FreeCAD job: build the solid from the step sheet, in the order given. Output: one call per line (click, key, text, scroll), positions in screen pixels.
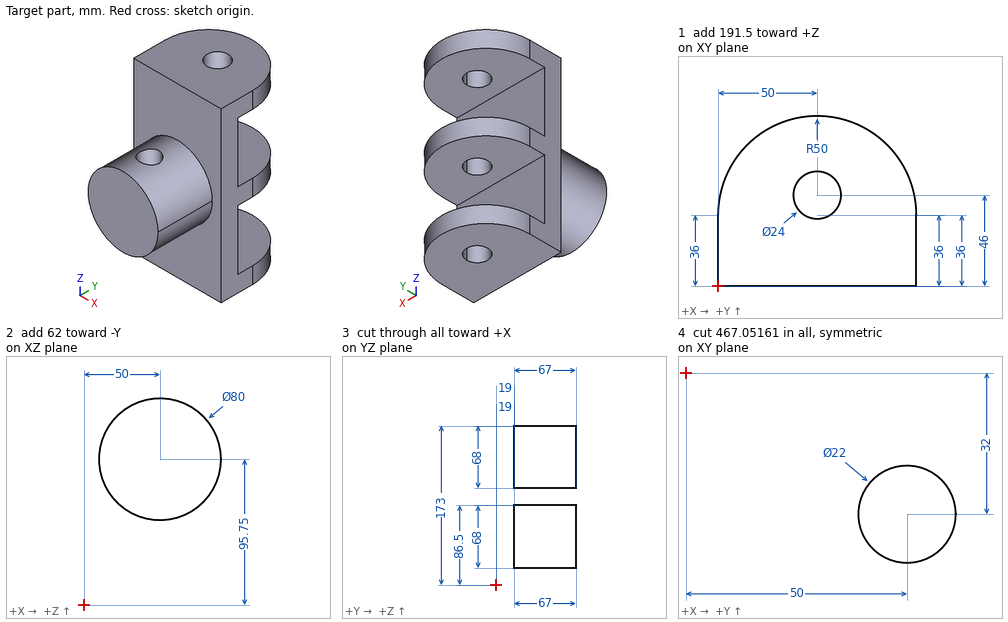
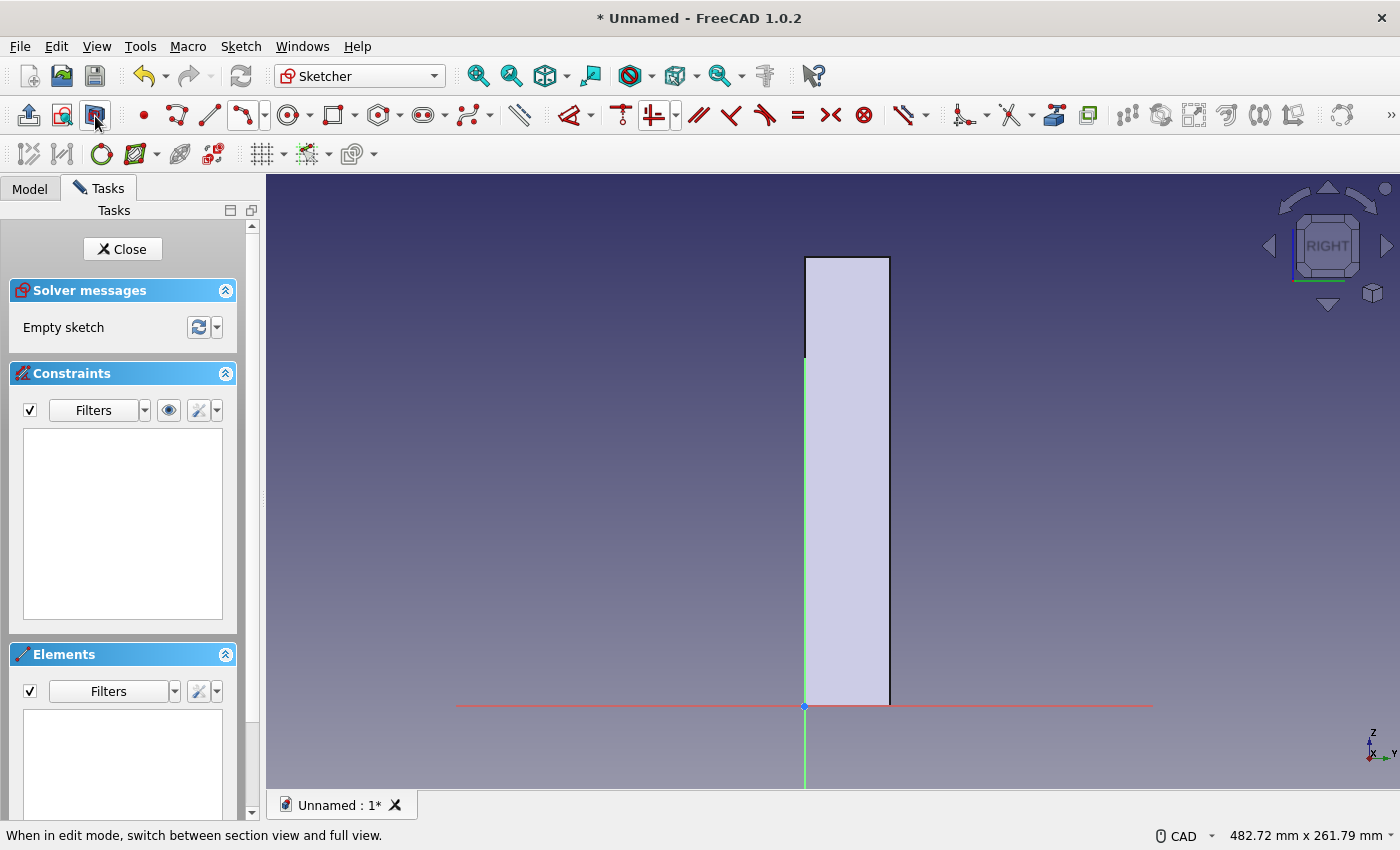
click(332, 116)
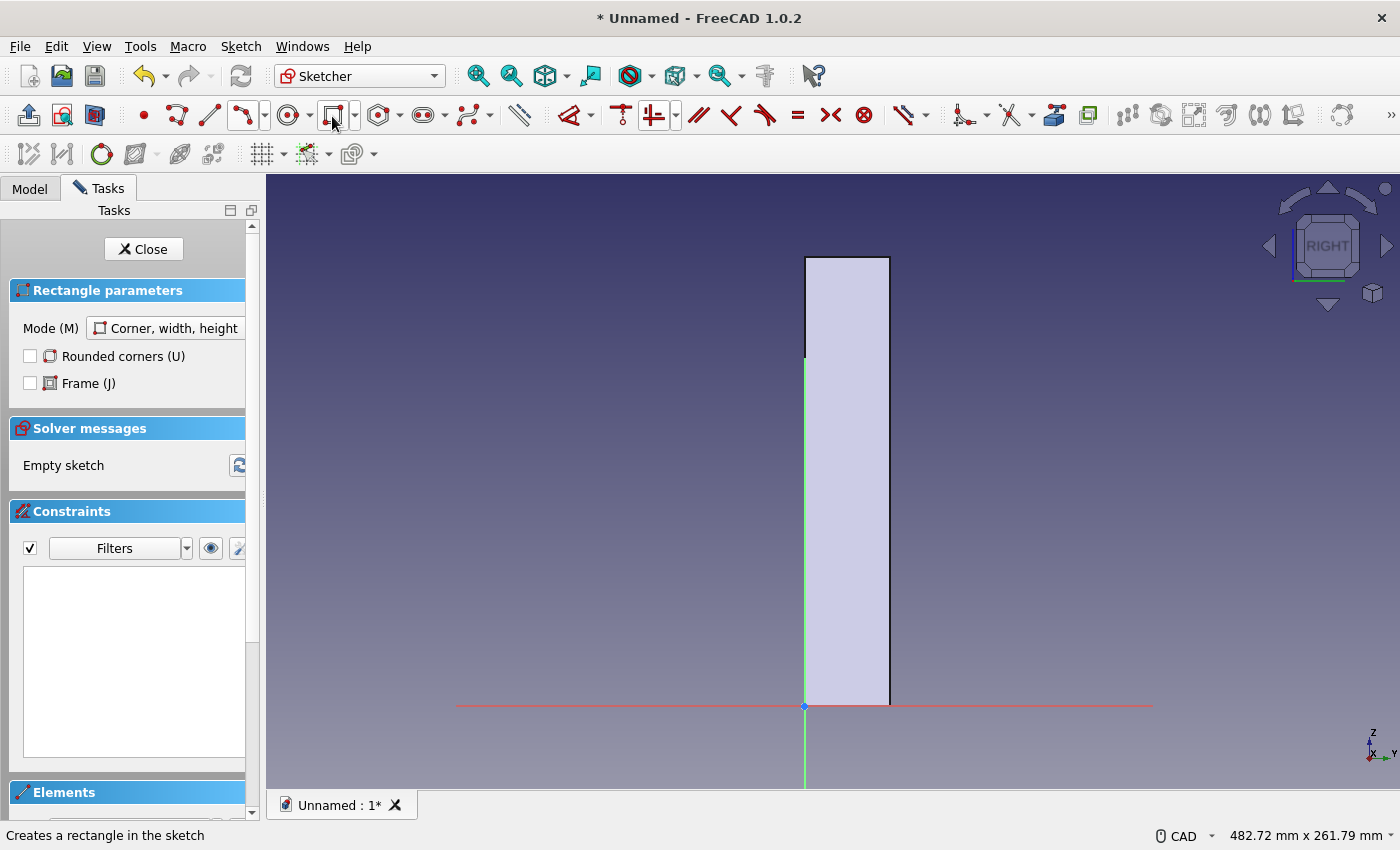
click(850, 503)
click(1007, 663)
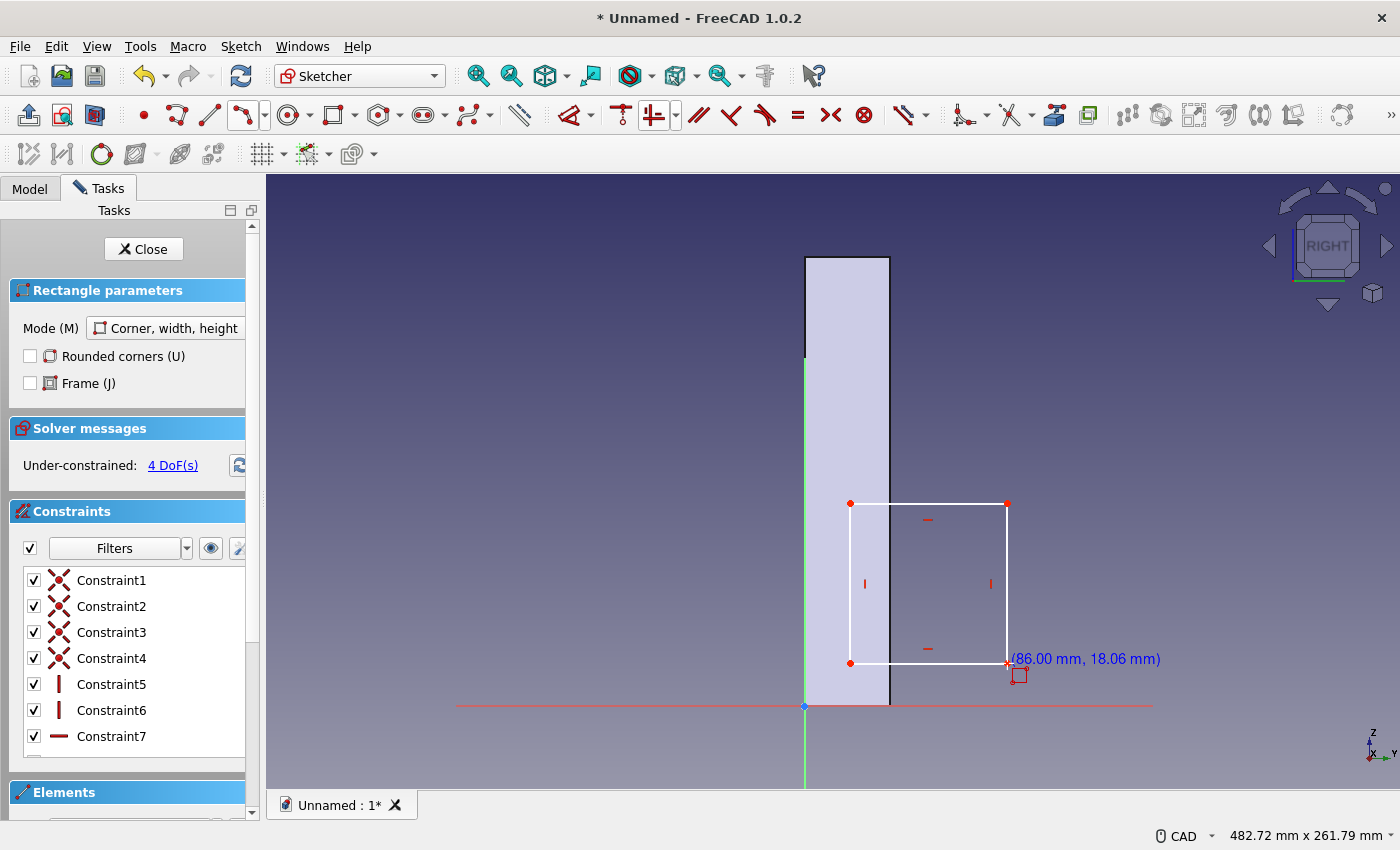
click(850, 300)
click(1007, 460)
key(Escape)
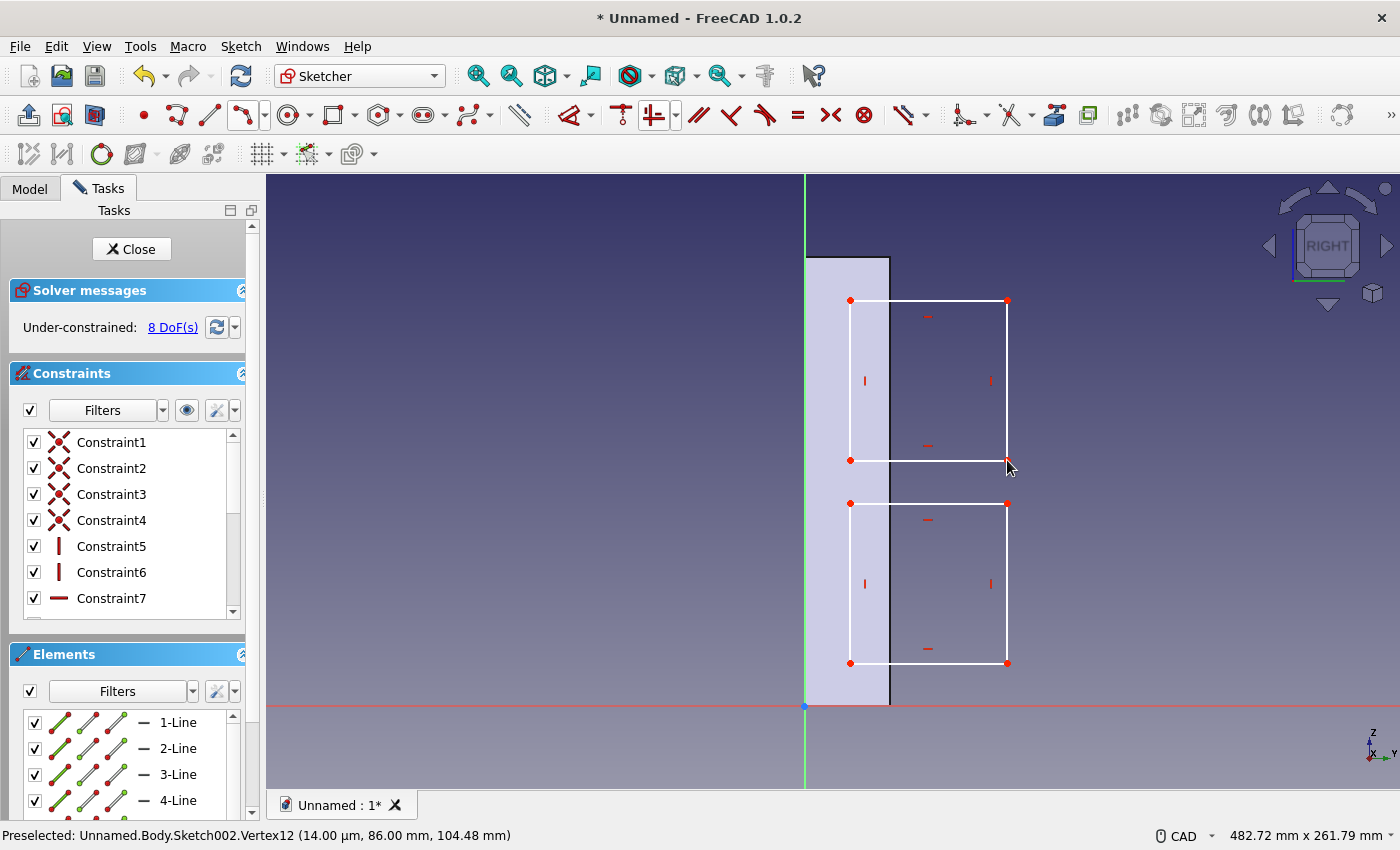
click(568, 116)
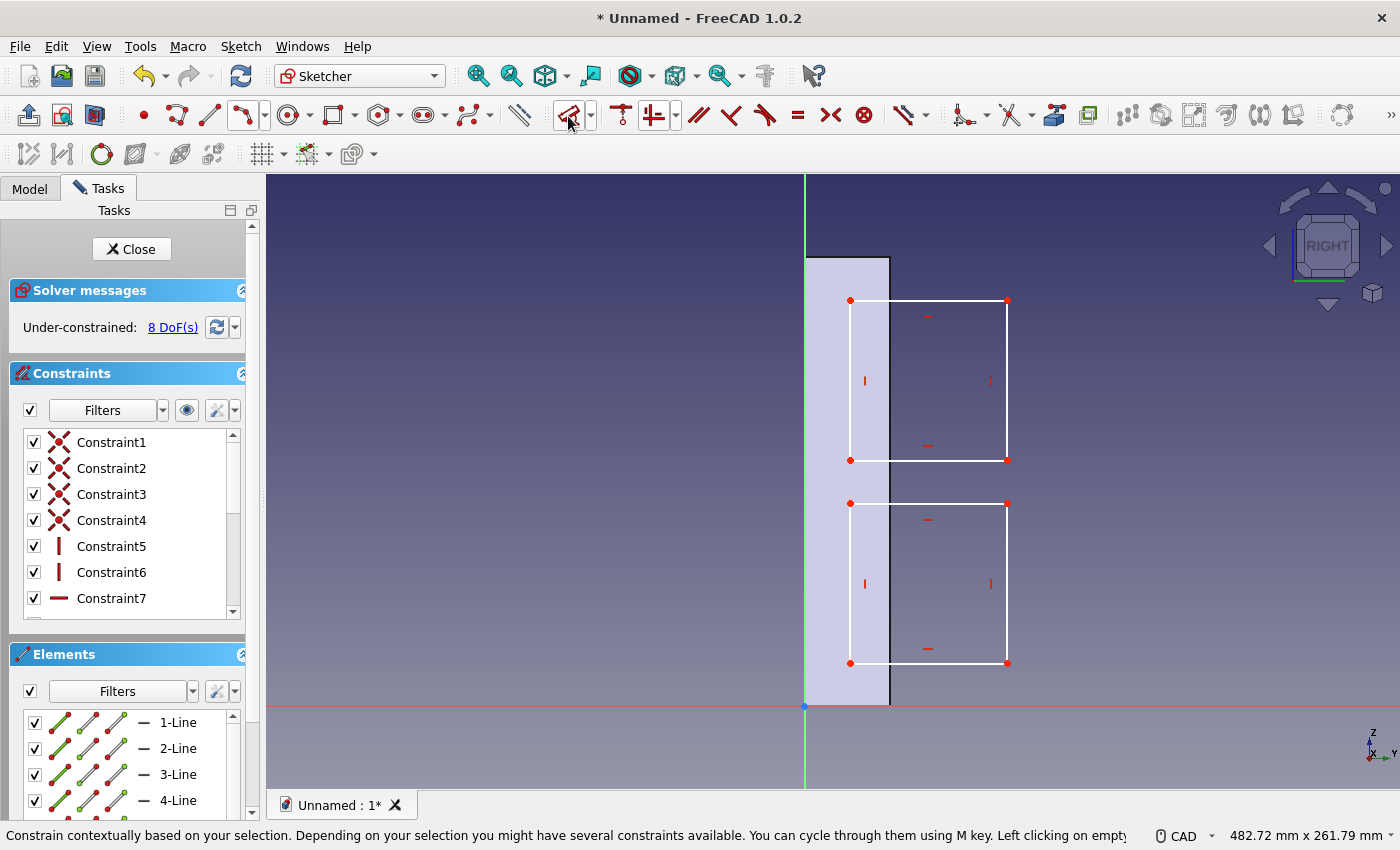
click(850, 552)
click(884, 584)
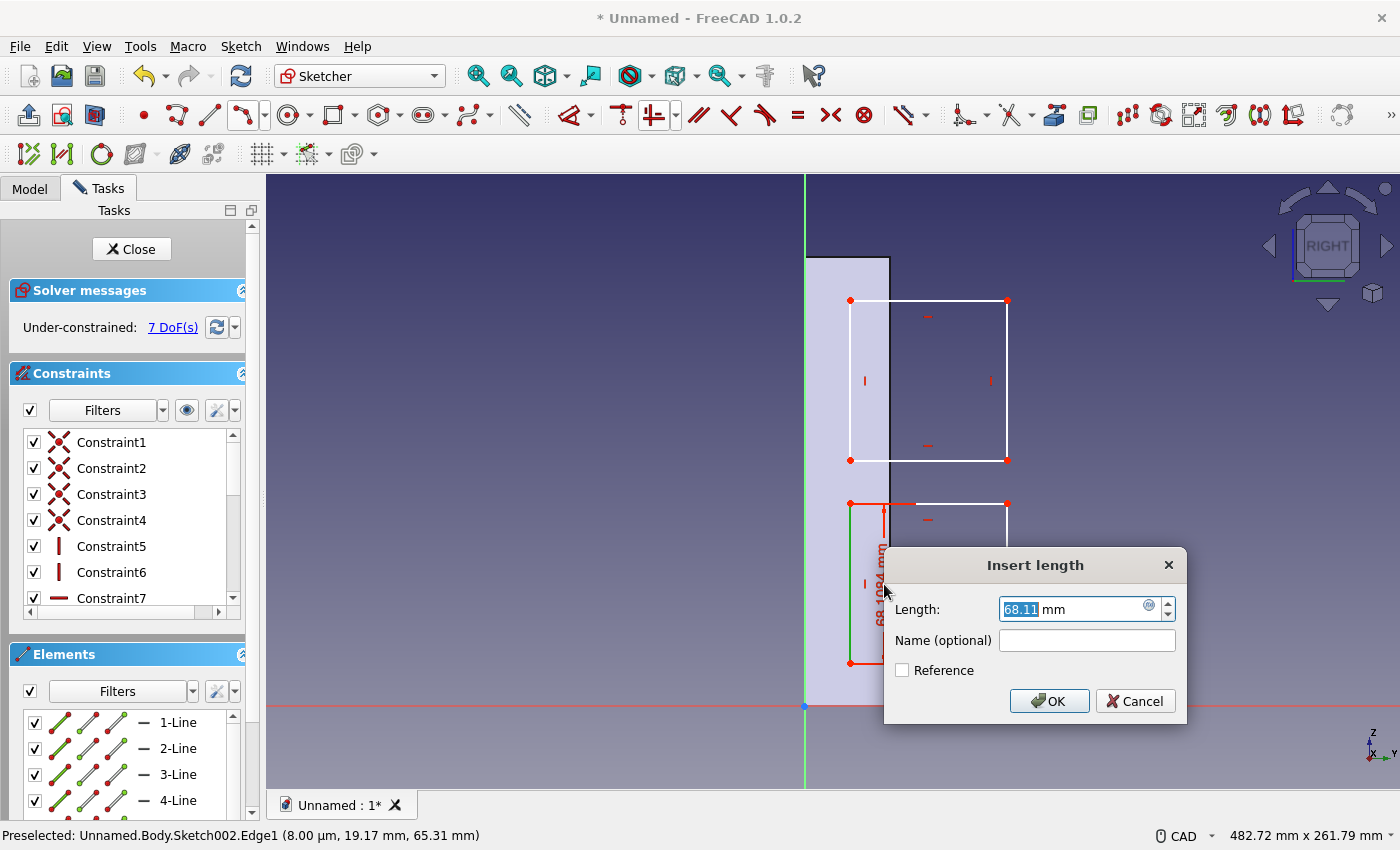
text(68)
key(Return)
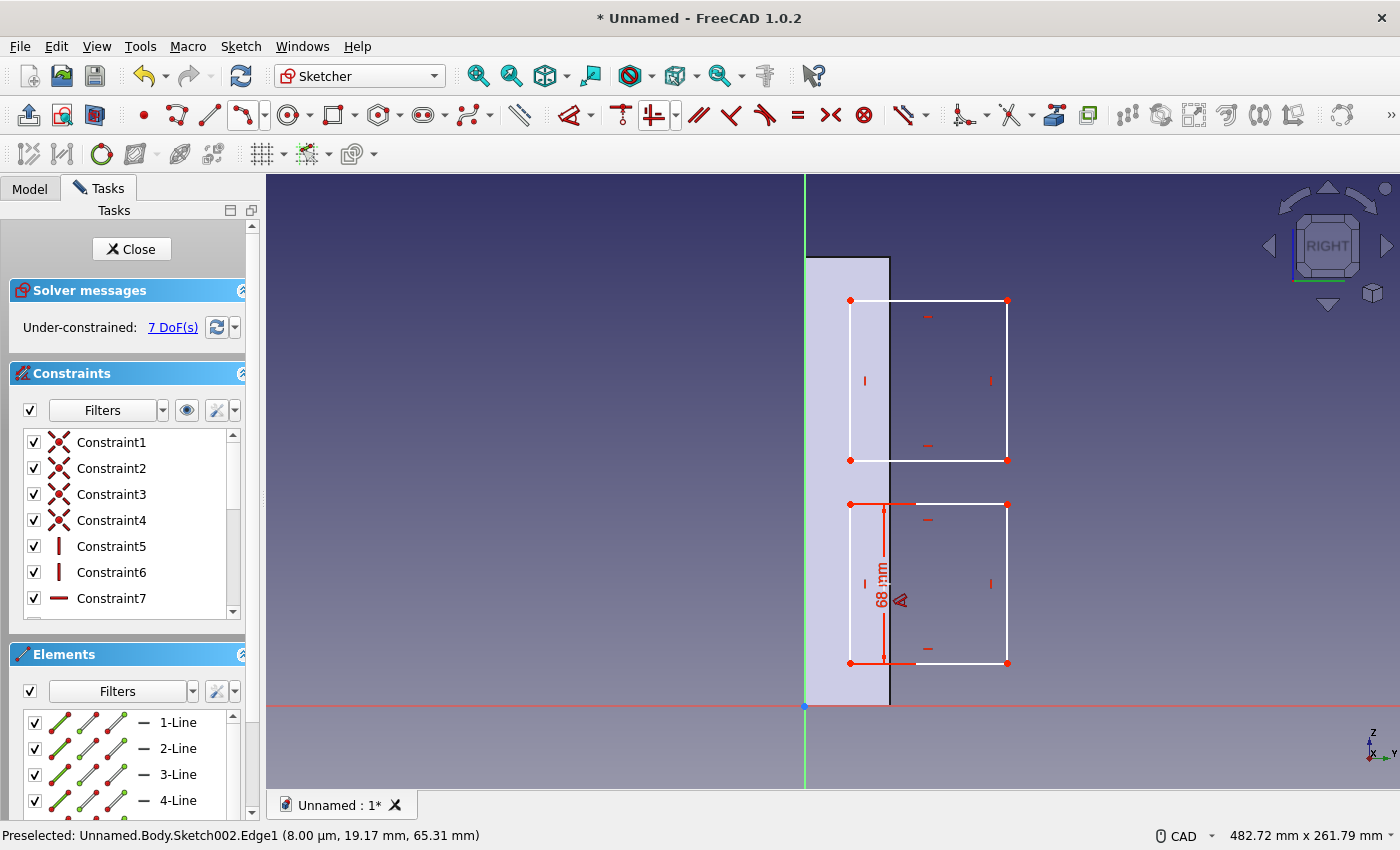
click(897, 664)
click(929, 630)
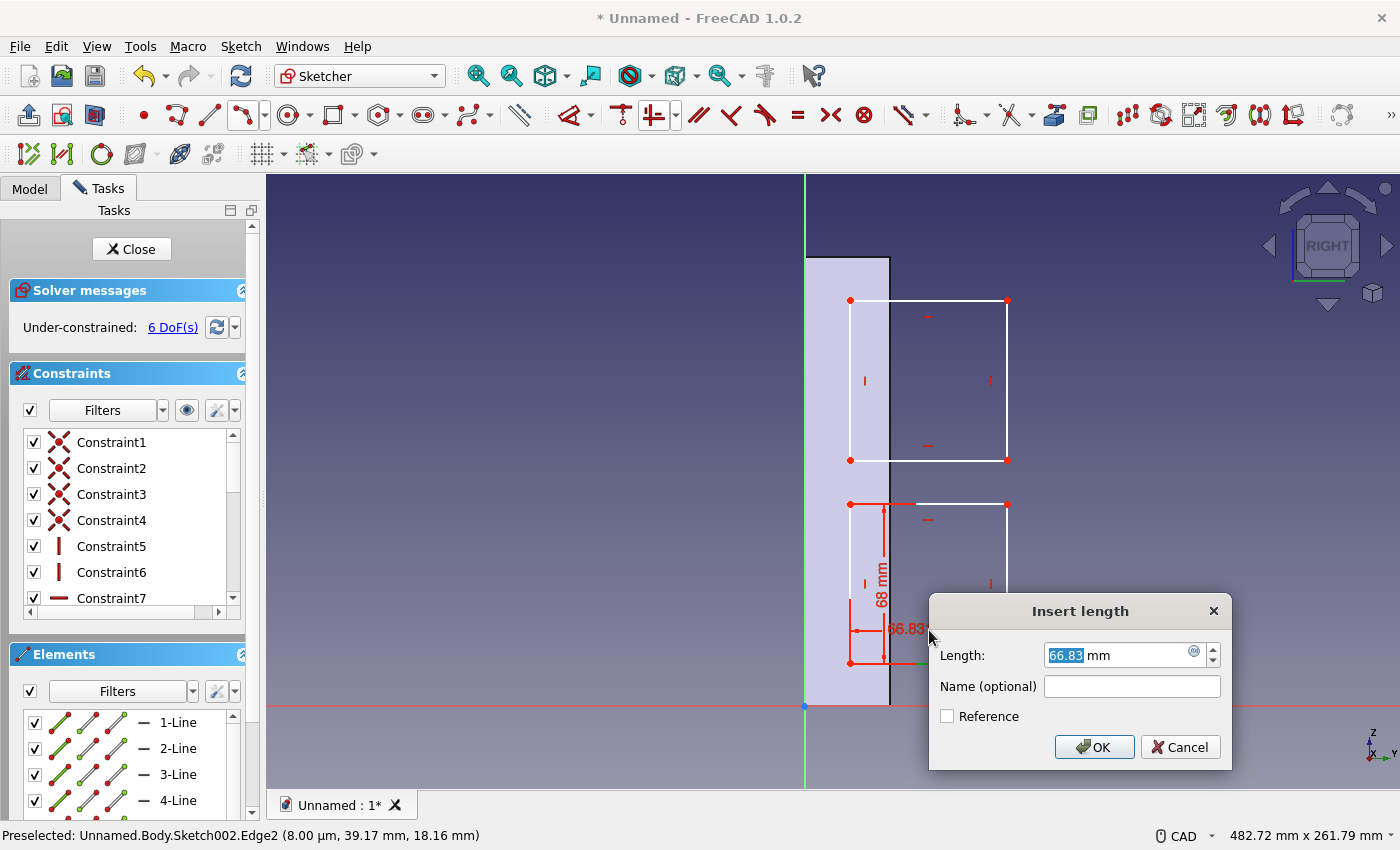
text(67)
key(Return)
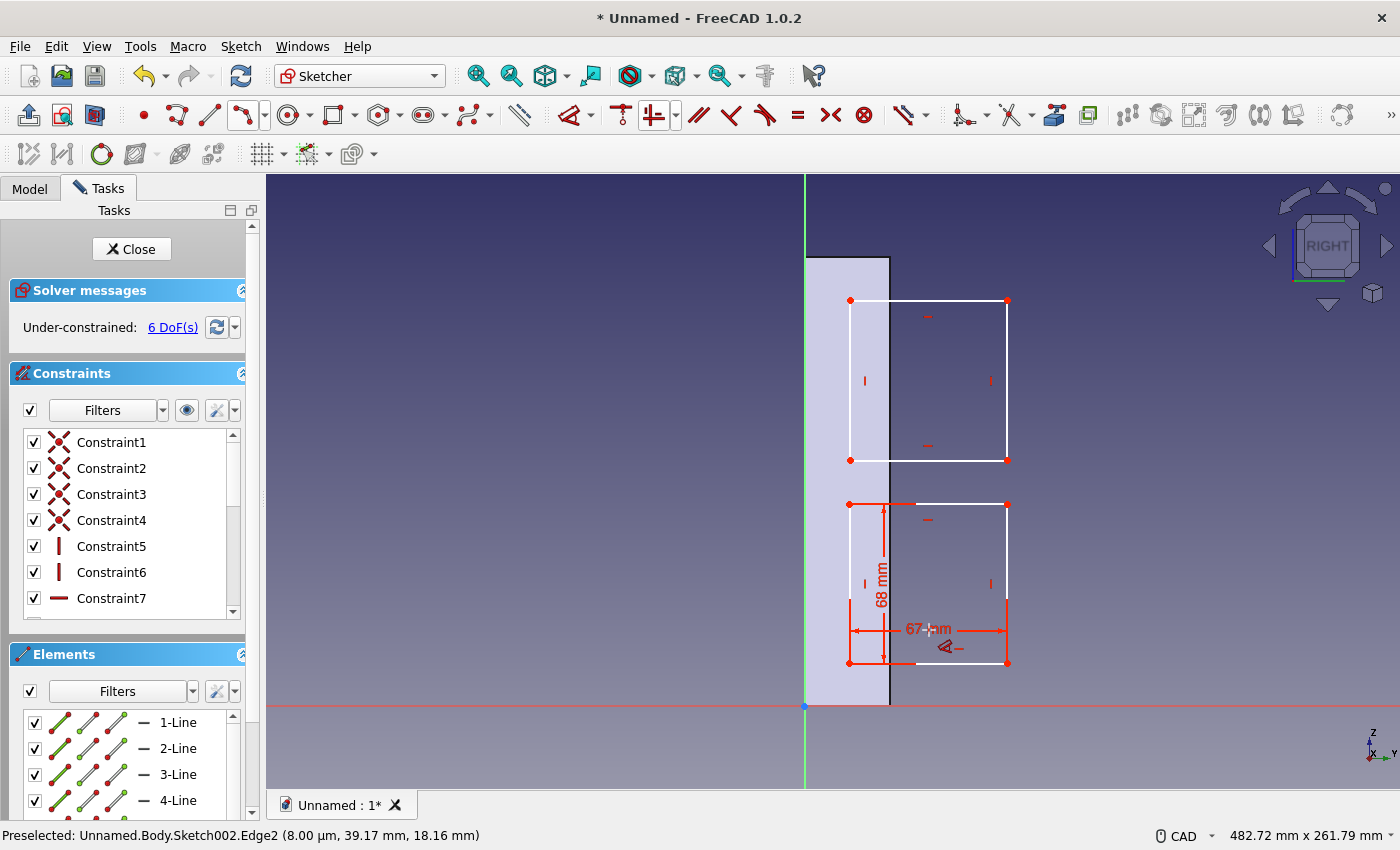
click(850, 349)
click(884, 381)